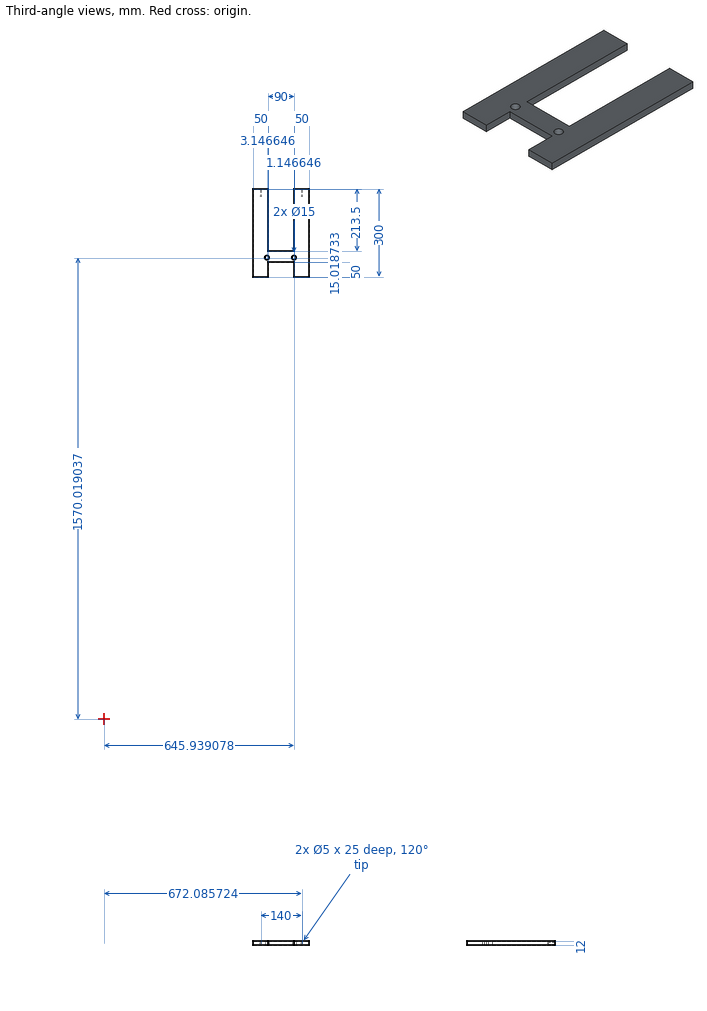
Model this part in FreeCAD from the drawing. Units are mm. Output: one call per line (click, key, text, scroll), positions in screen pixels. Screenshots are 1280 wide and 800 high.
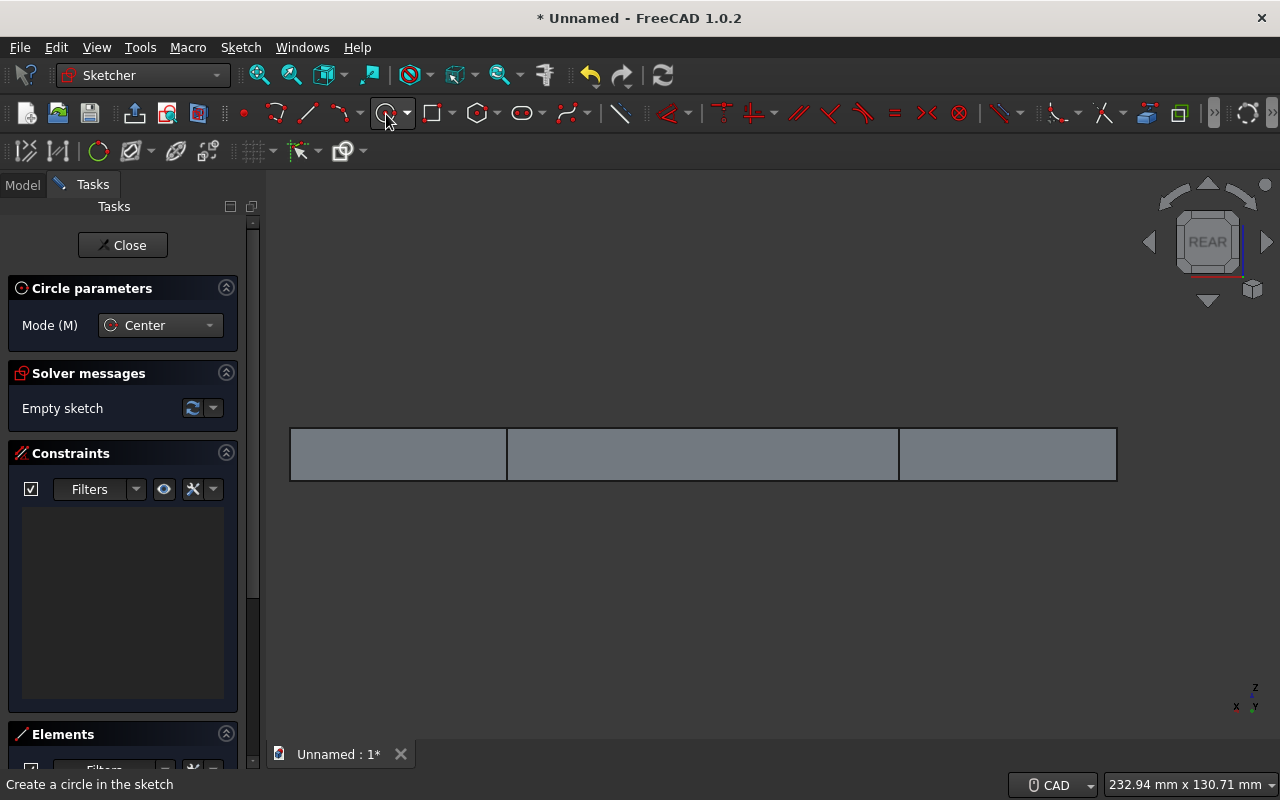
scroll(399, 454, up, 4)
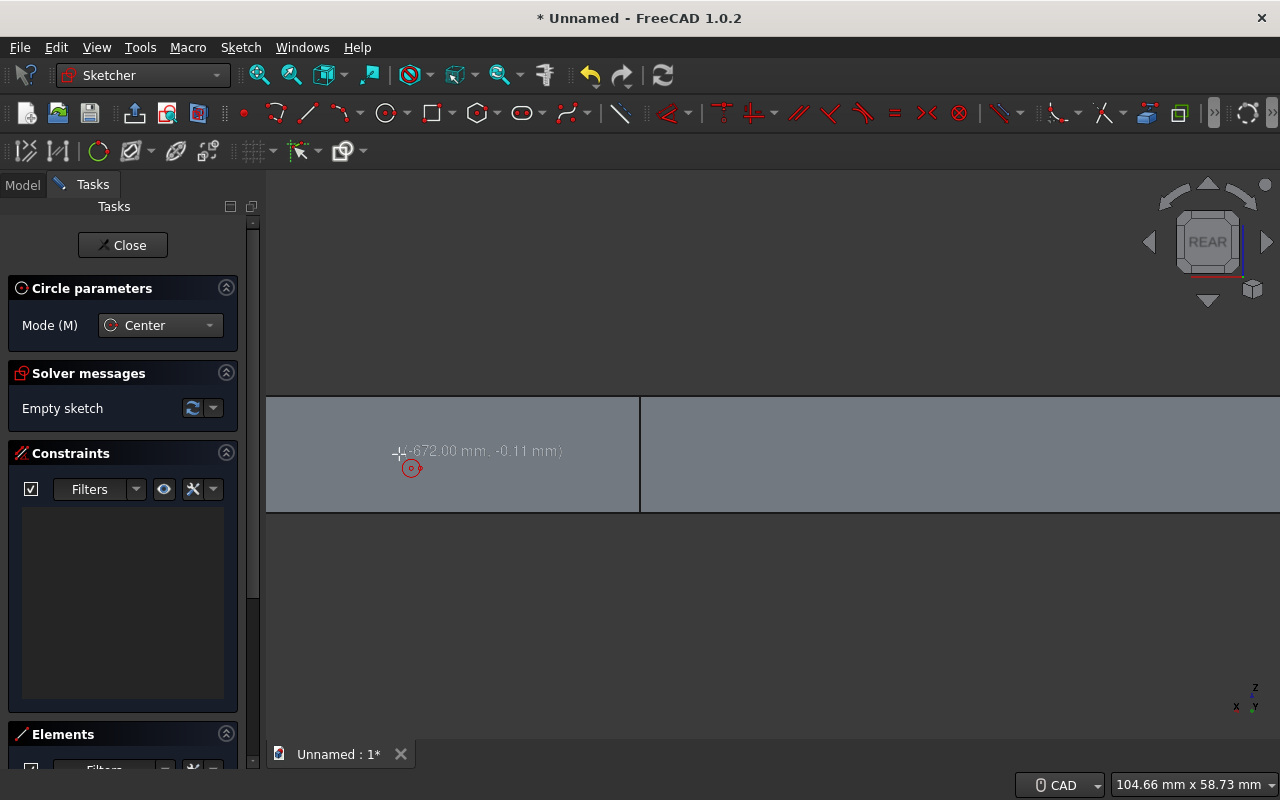
click(398, 454)
move(415, 437)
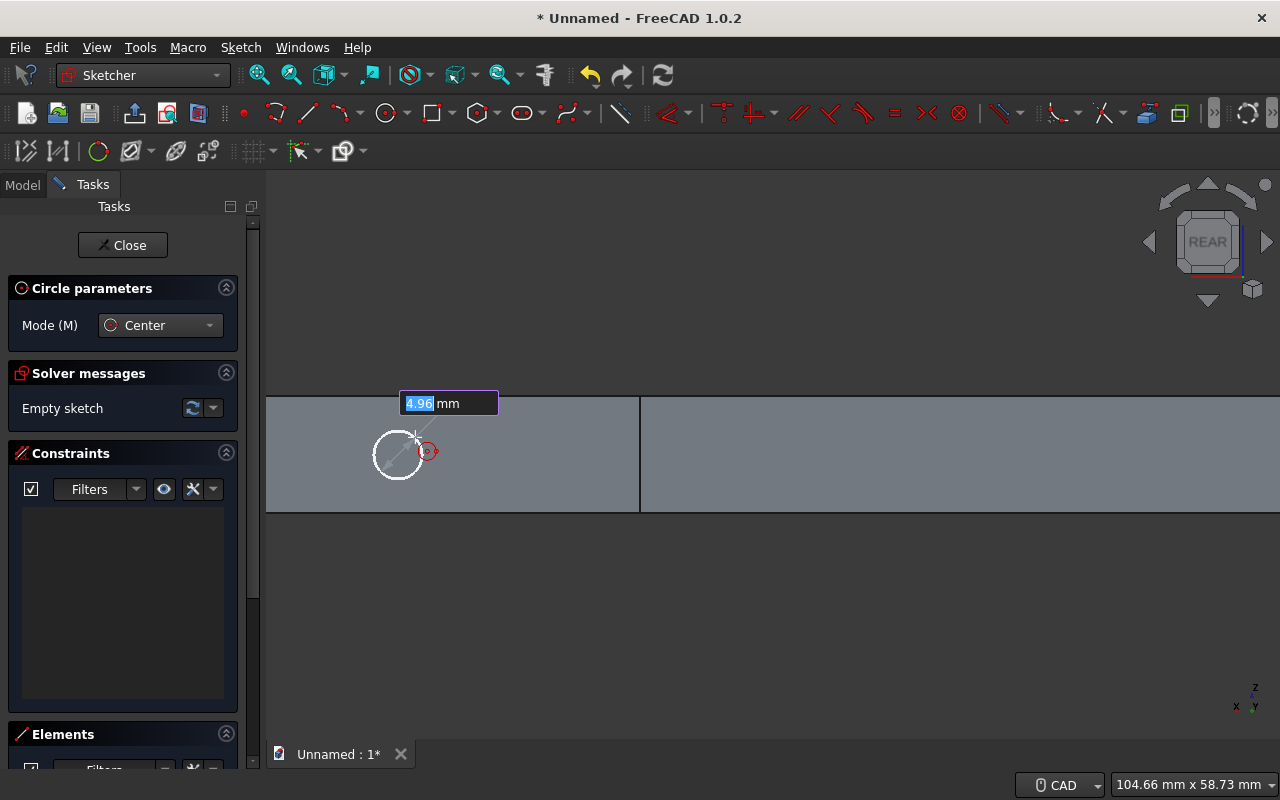
text(5)
key(Return)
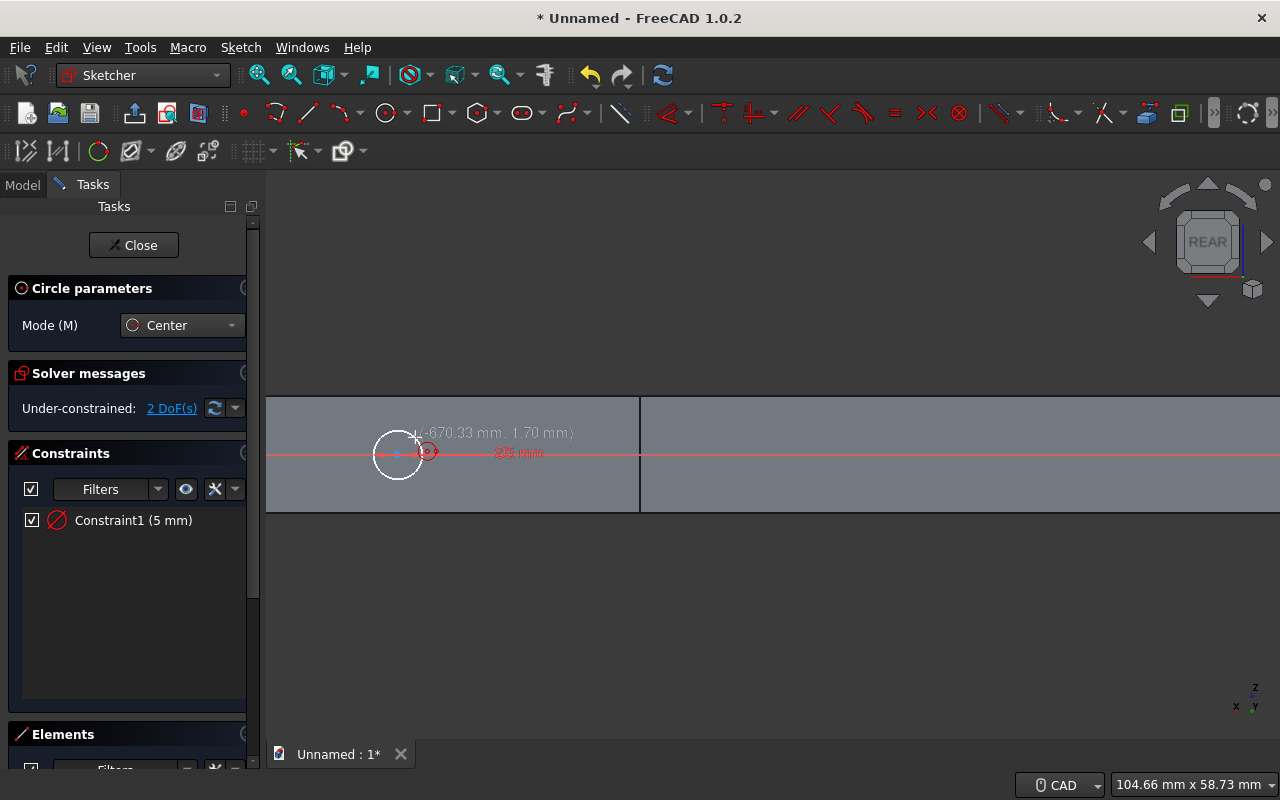
scroll(401, 454, down, 4)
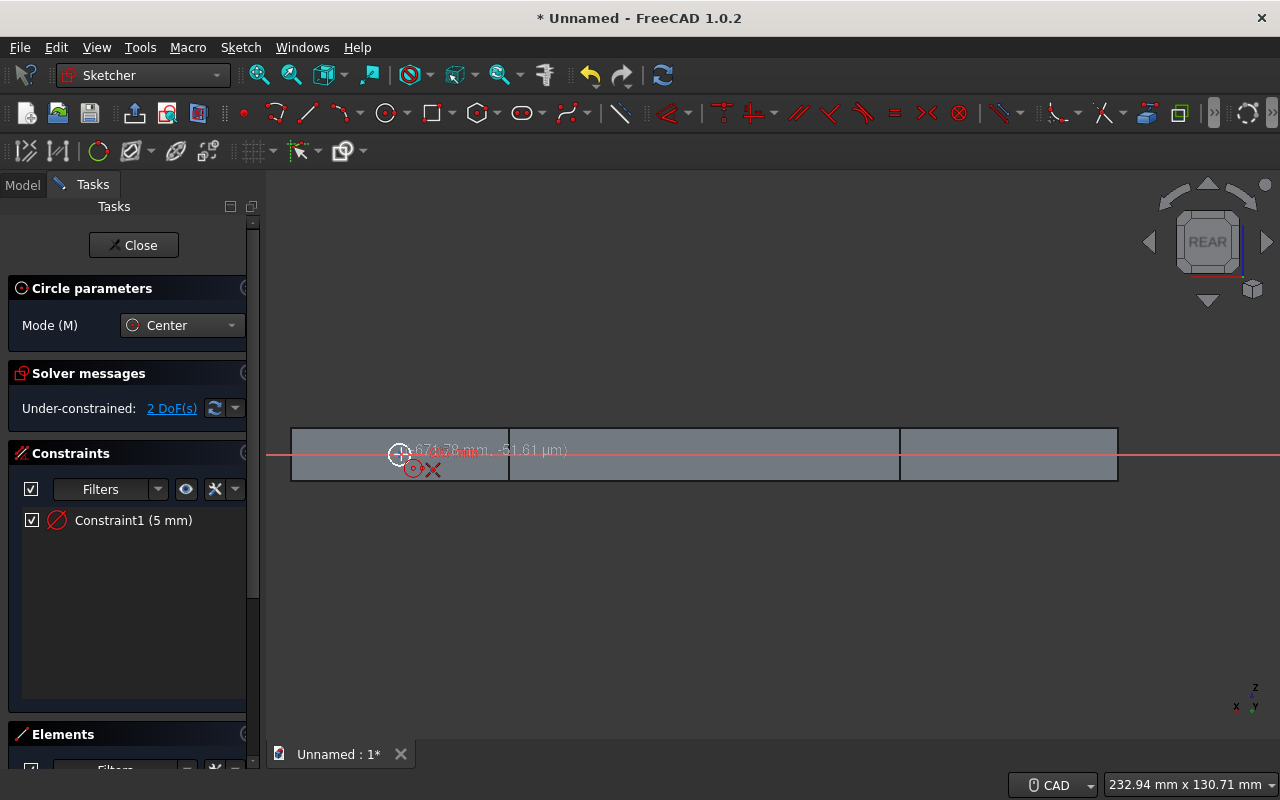
scroll(1009, 454, up, 4)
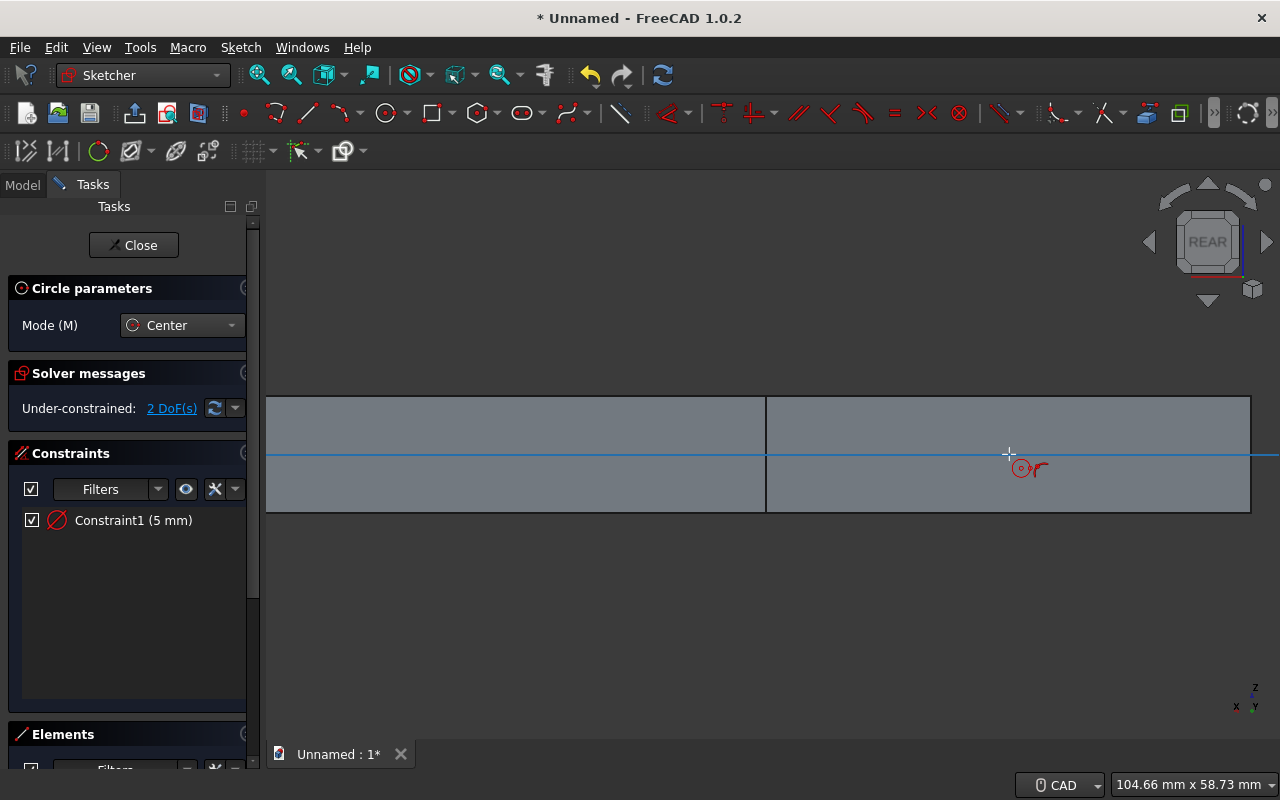
click(1008, 454)
move(1026, 437)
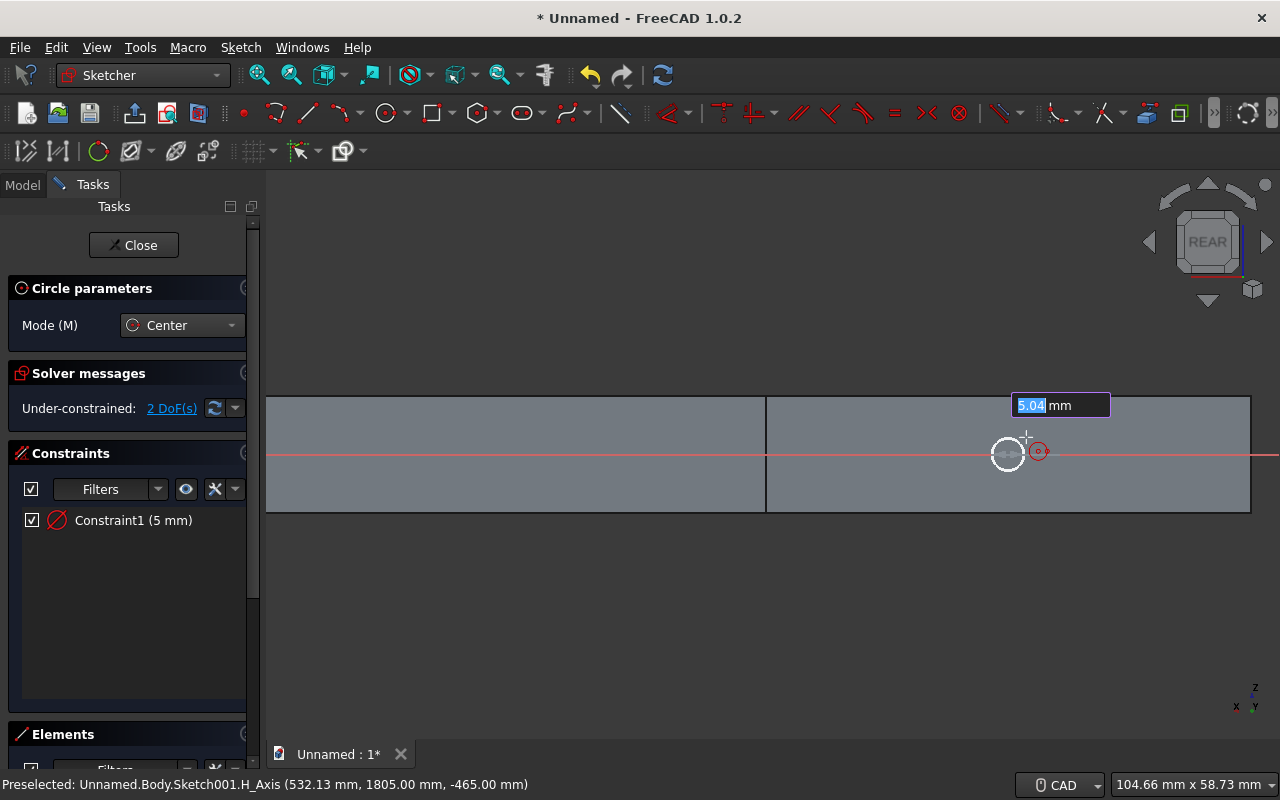
text(5)
key(Return)
key(Escape)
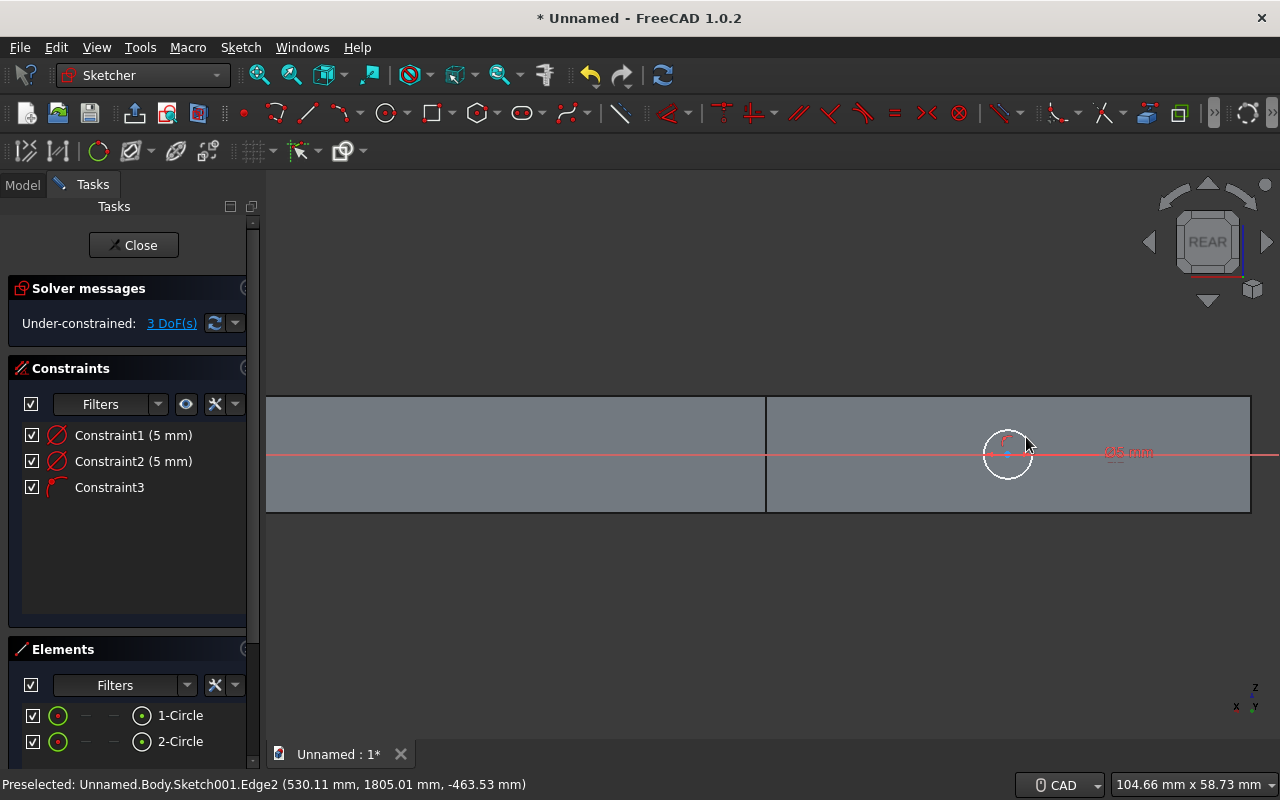
scroll(1010, 454, down, 4)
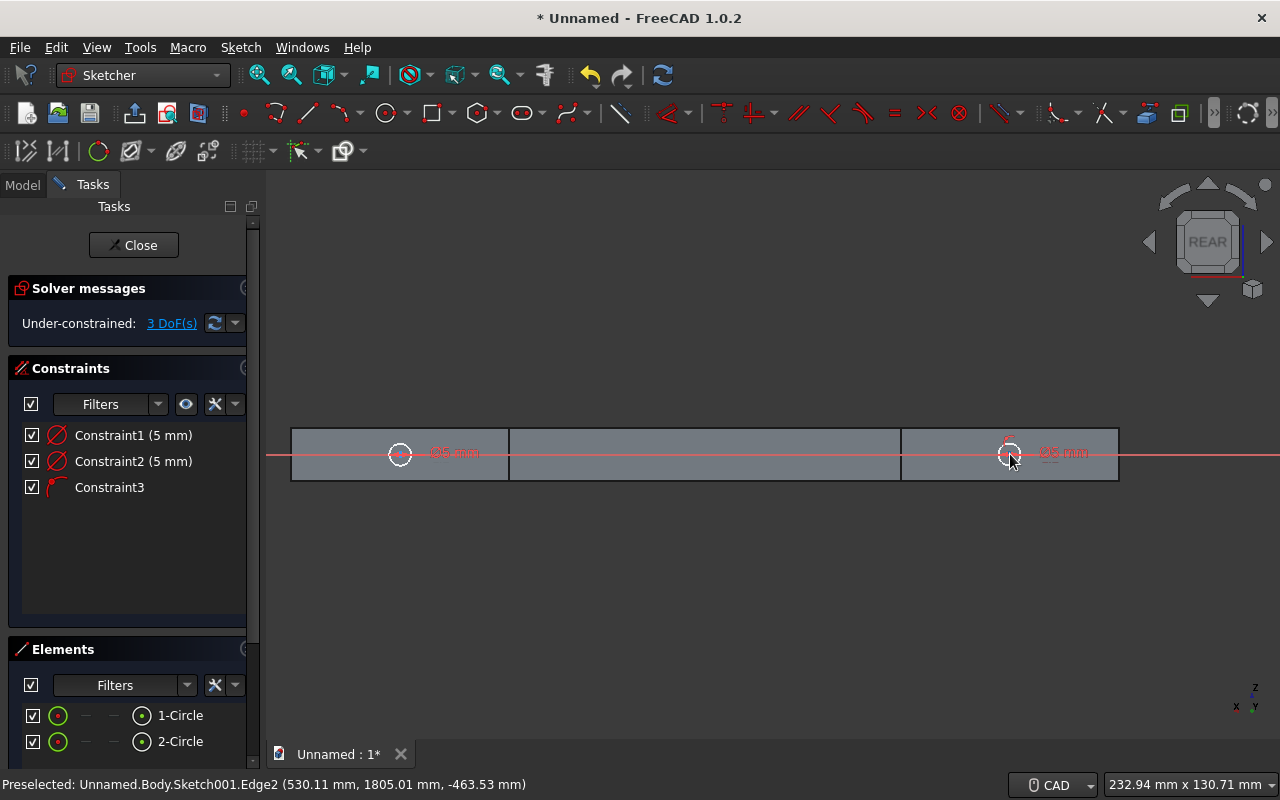
click(400, 455)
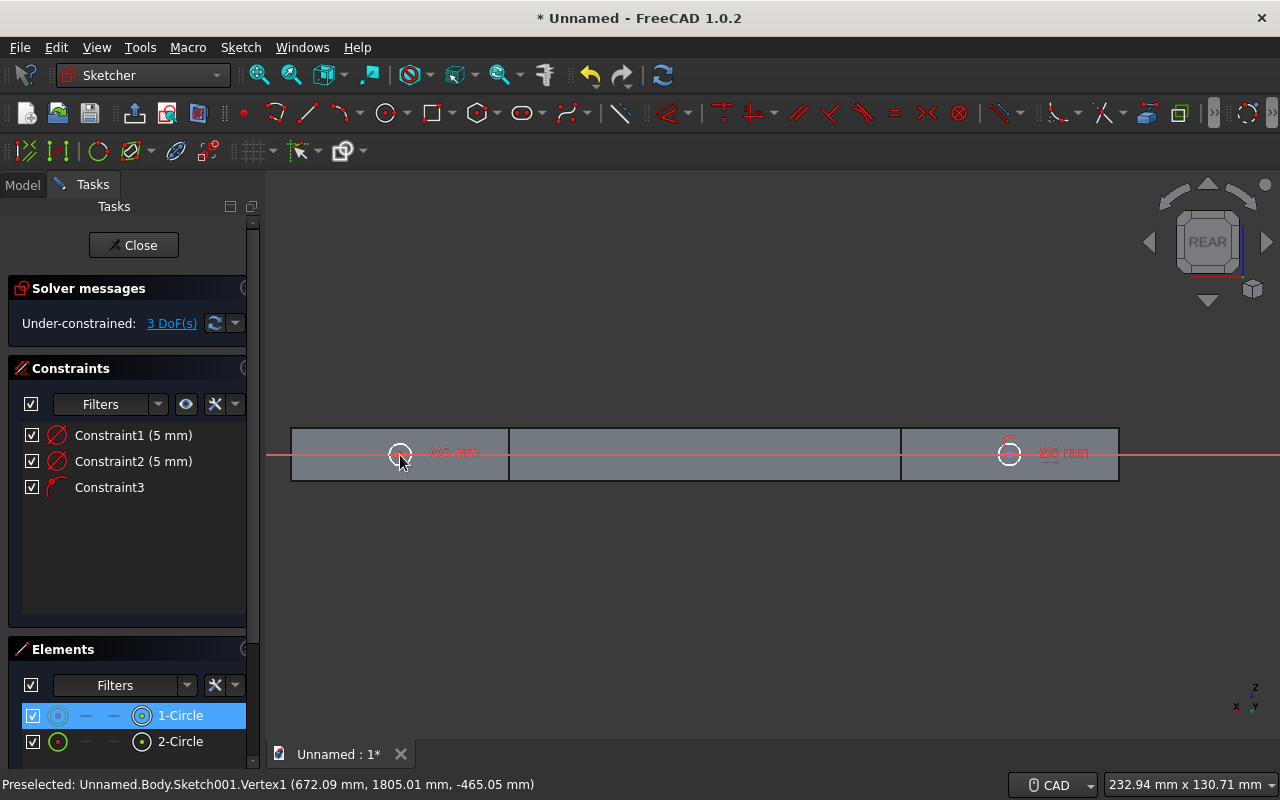
click(353, 454)